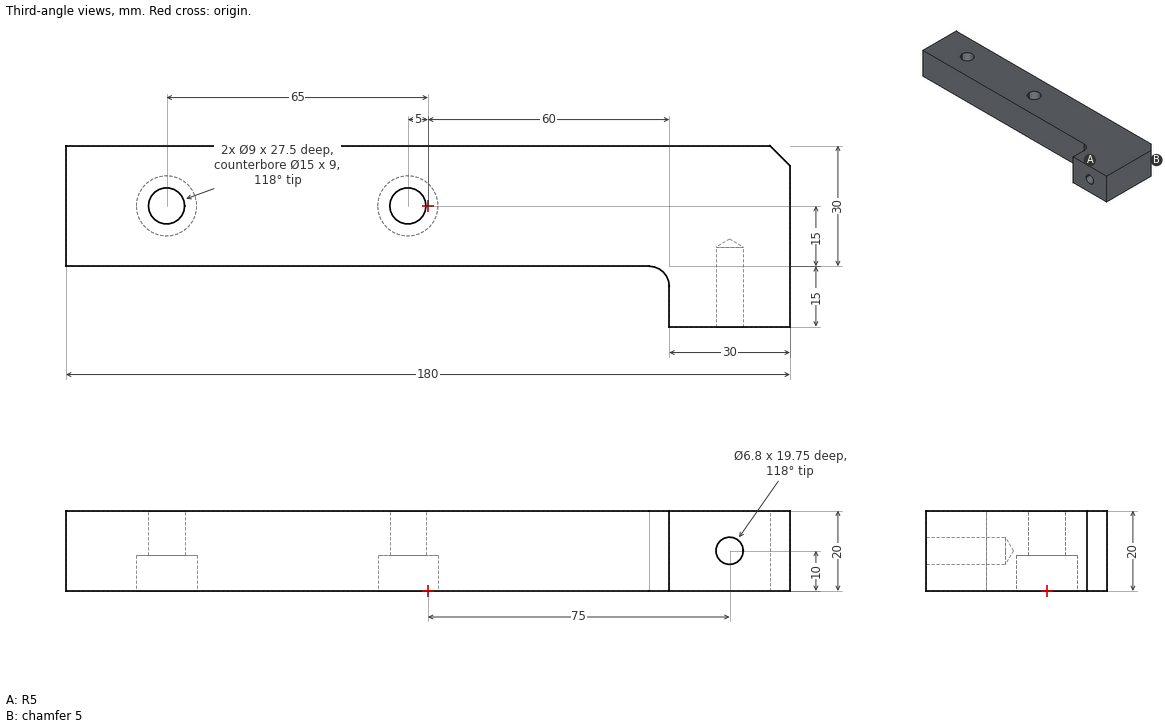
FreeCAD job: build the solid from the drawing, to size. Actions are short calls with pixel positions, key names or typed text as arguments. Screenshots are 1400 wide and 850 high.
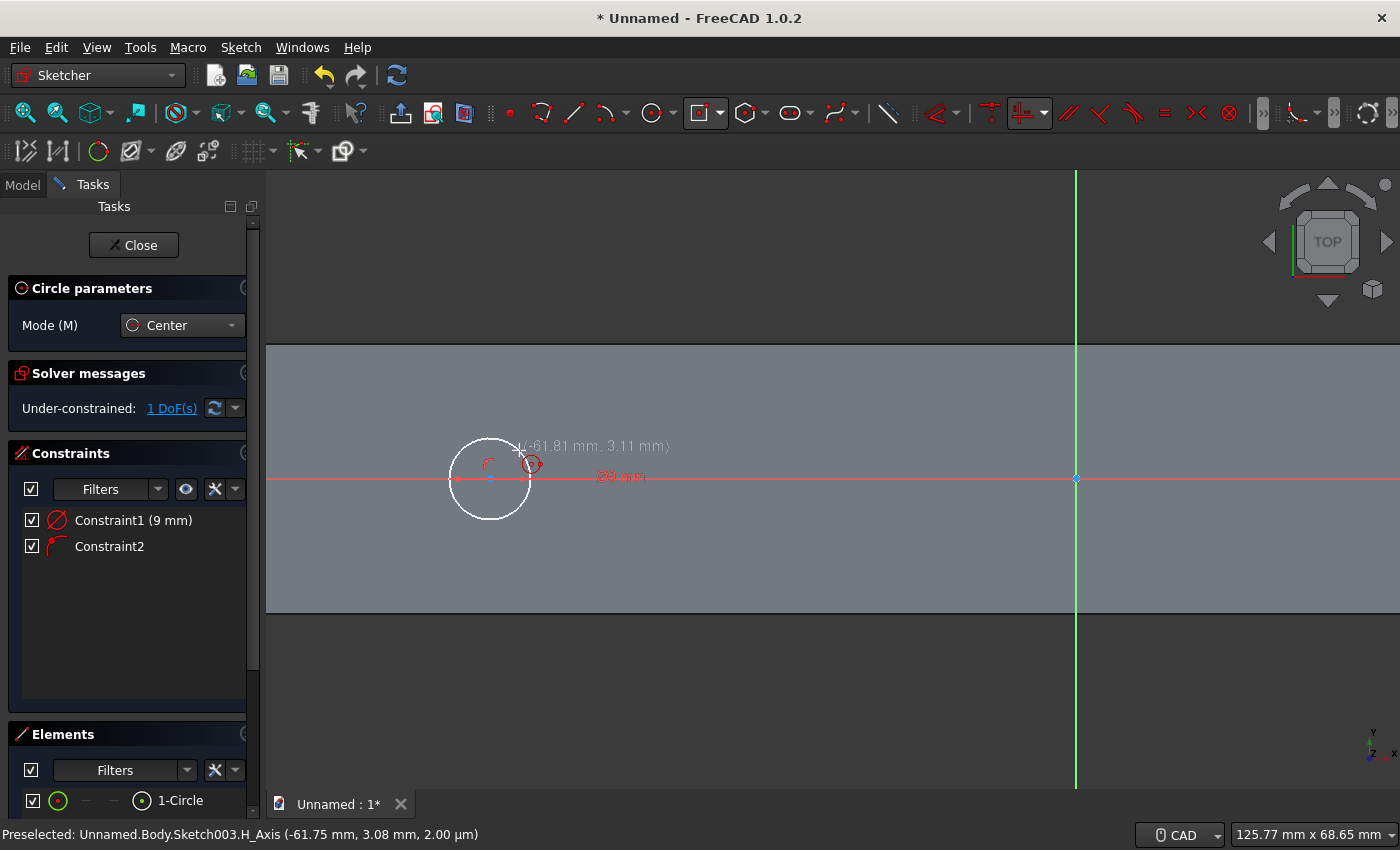
click(1031, 479)
move(1060, 450)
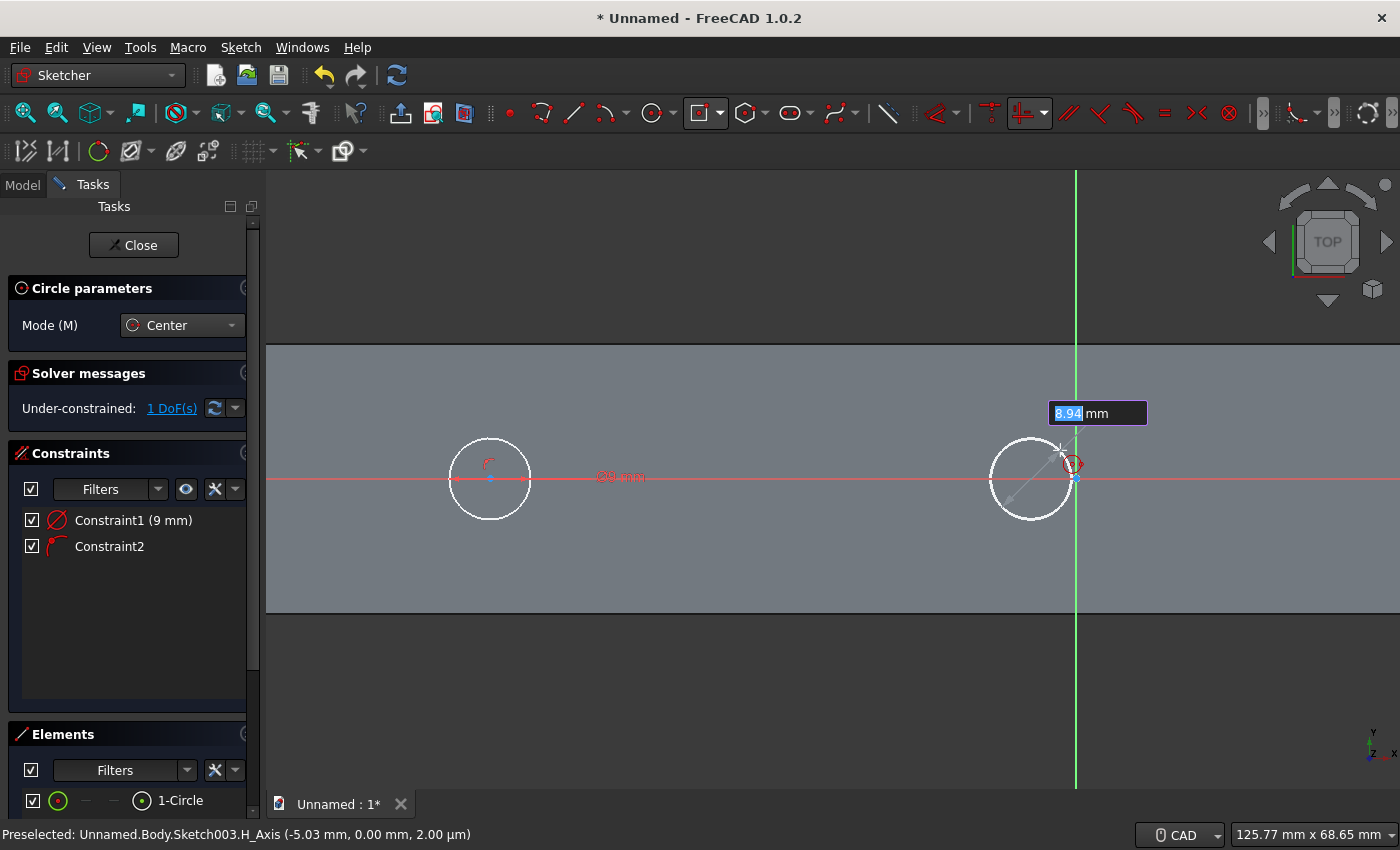
text(9)
key(Return)
key(Escape)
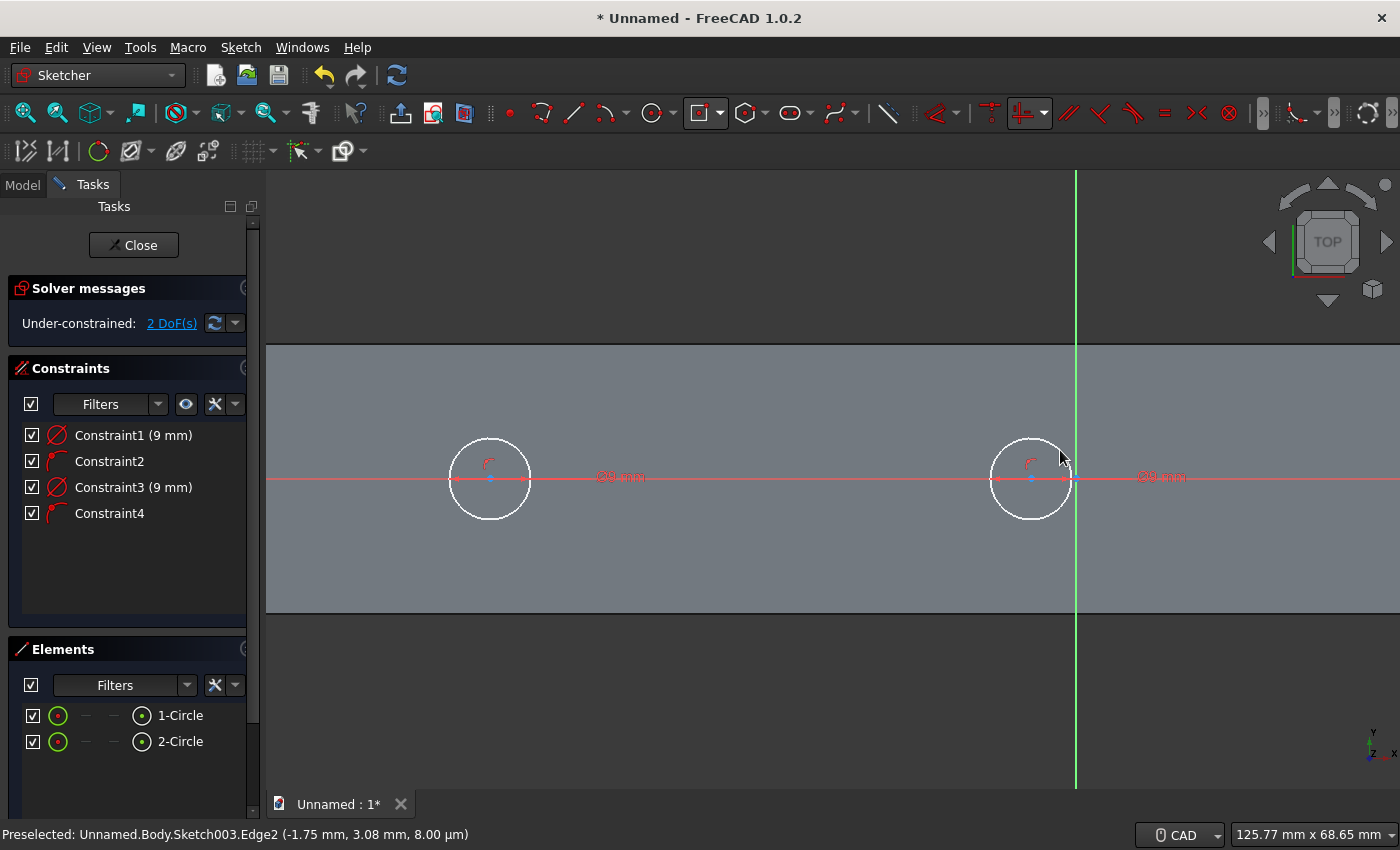
click(936, 114)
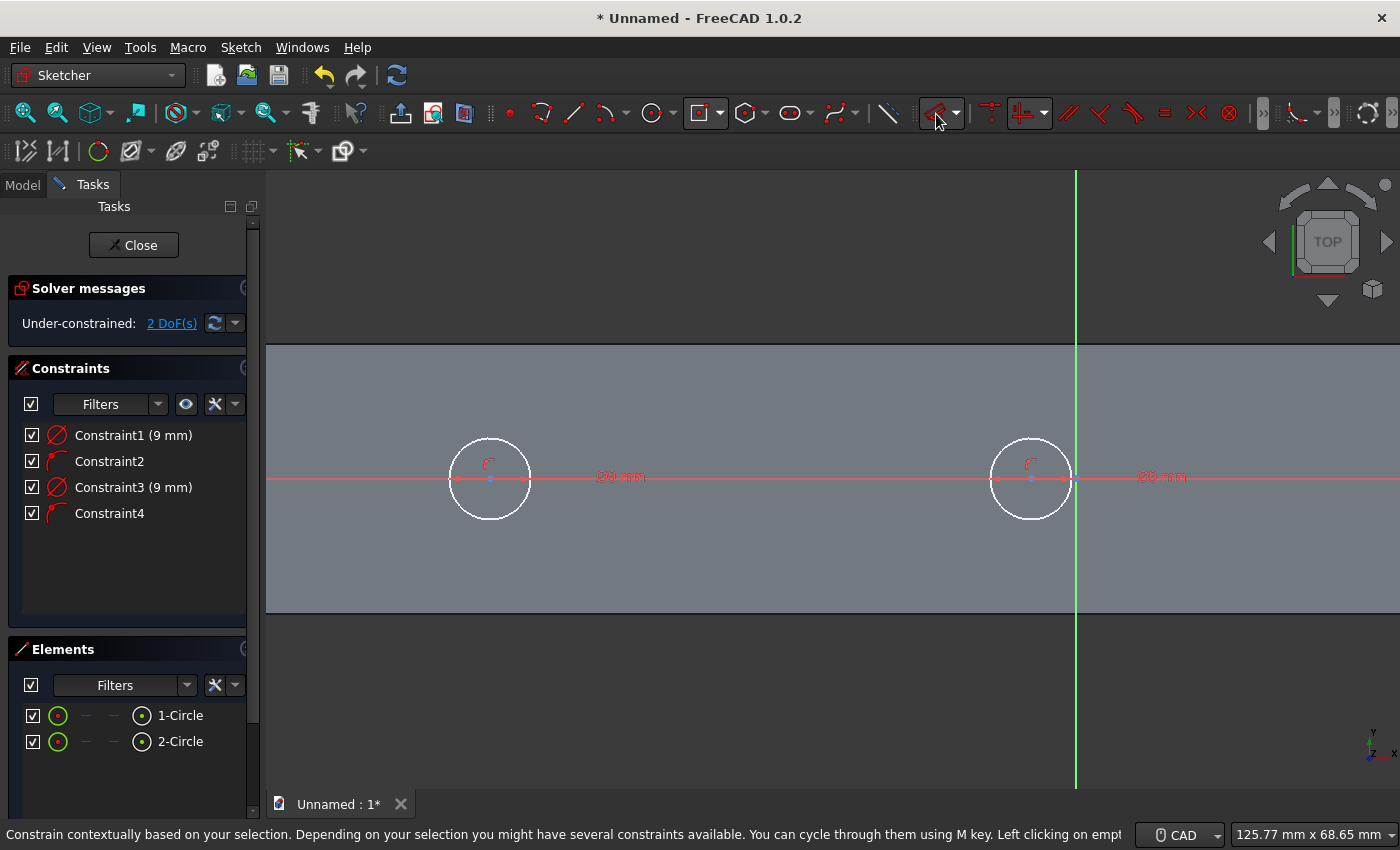
click(1031, 479)
click(1054, 537)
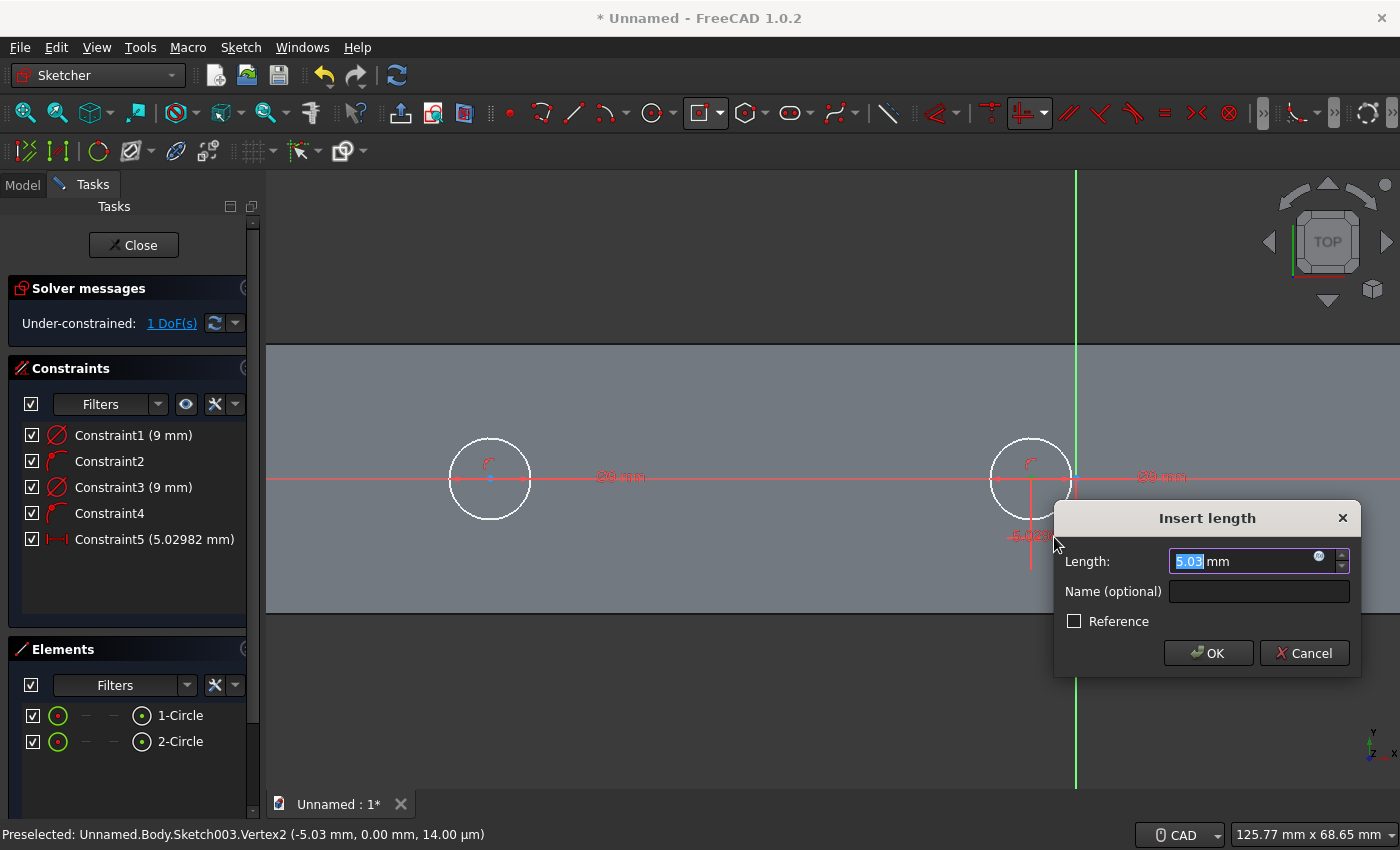
text(5)
key(Return)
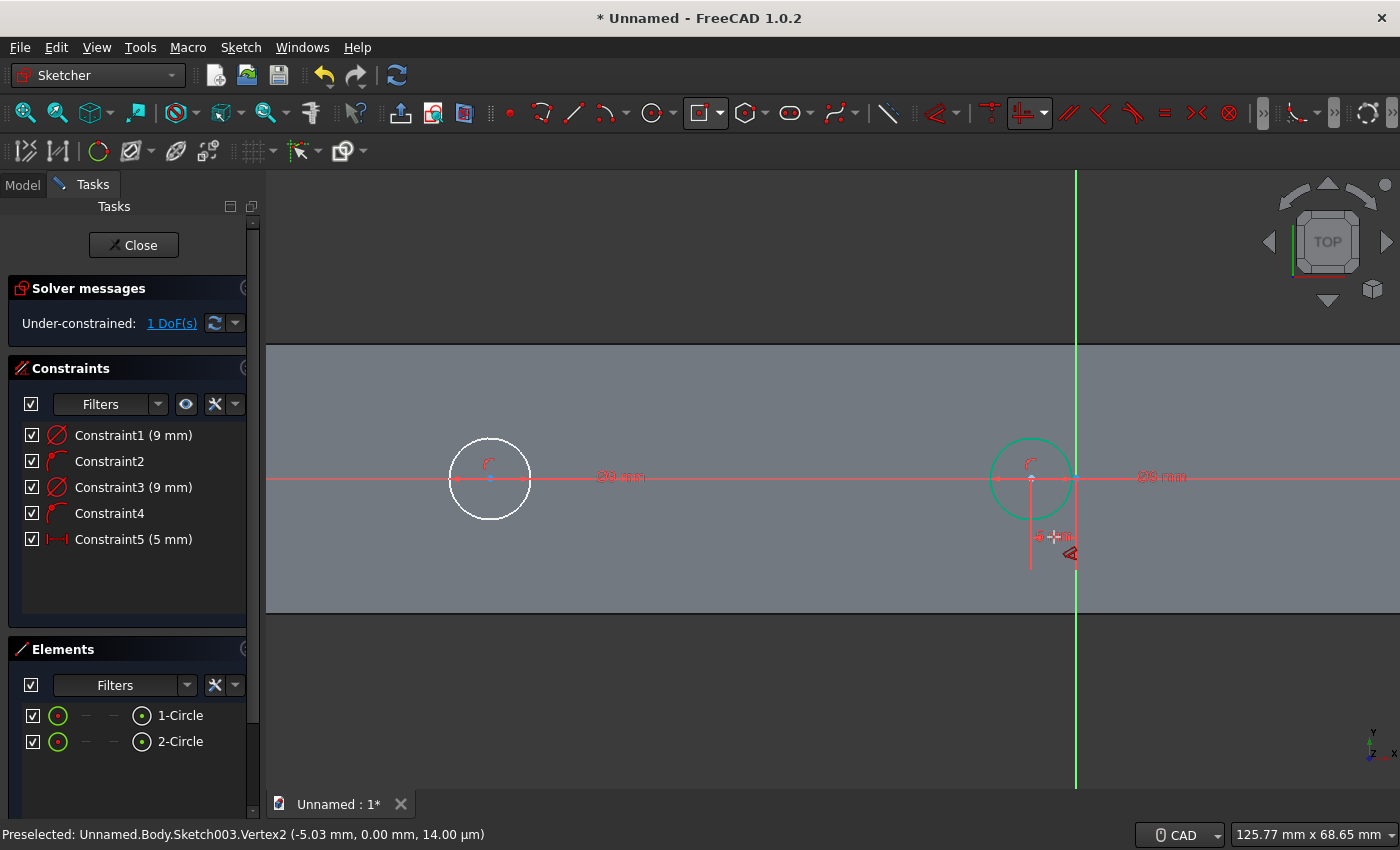
click(490, 479)
click(783, 513)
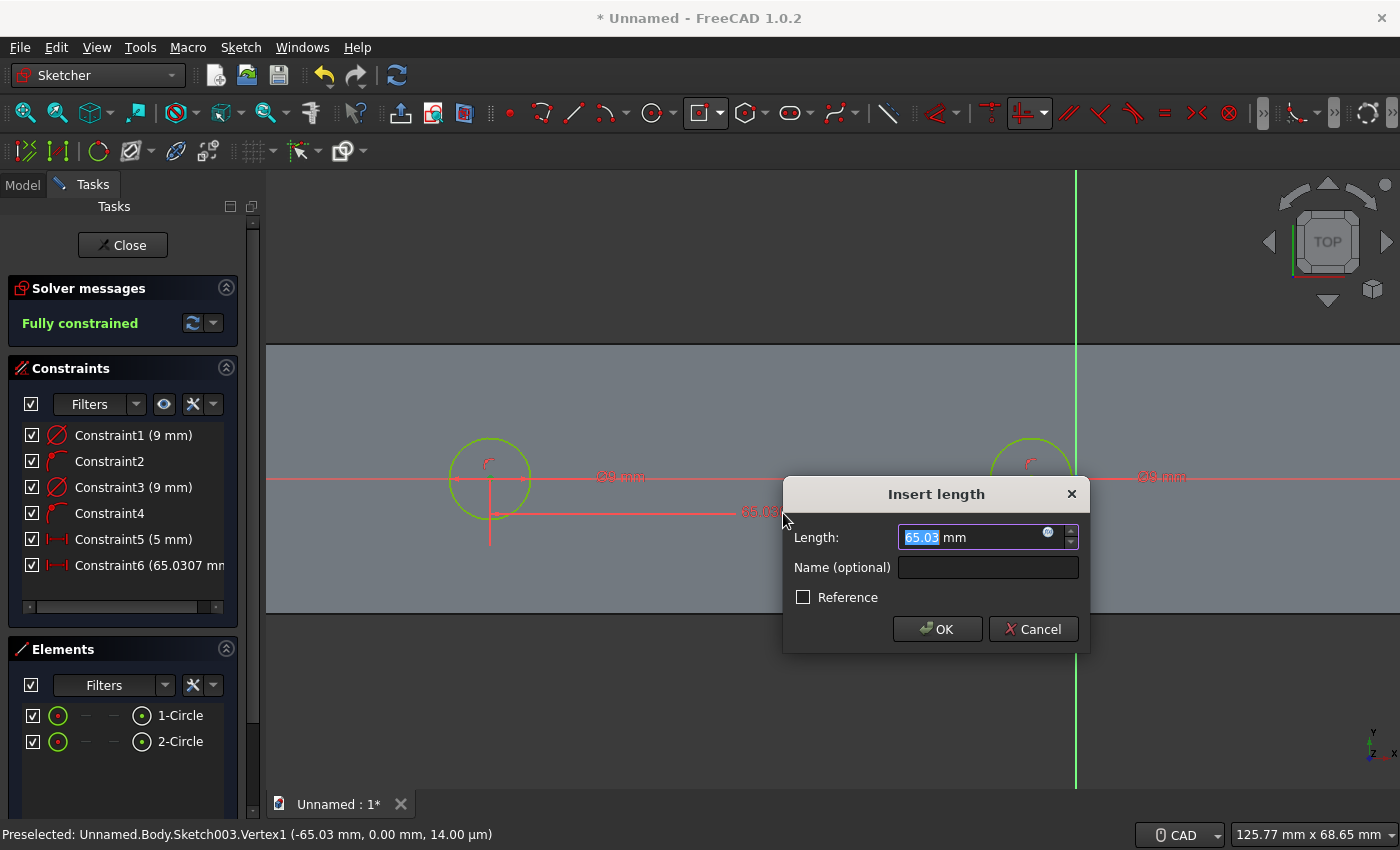
text(65)
key(Return)
key(Escape)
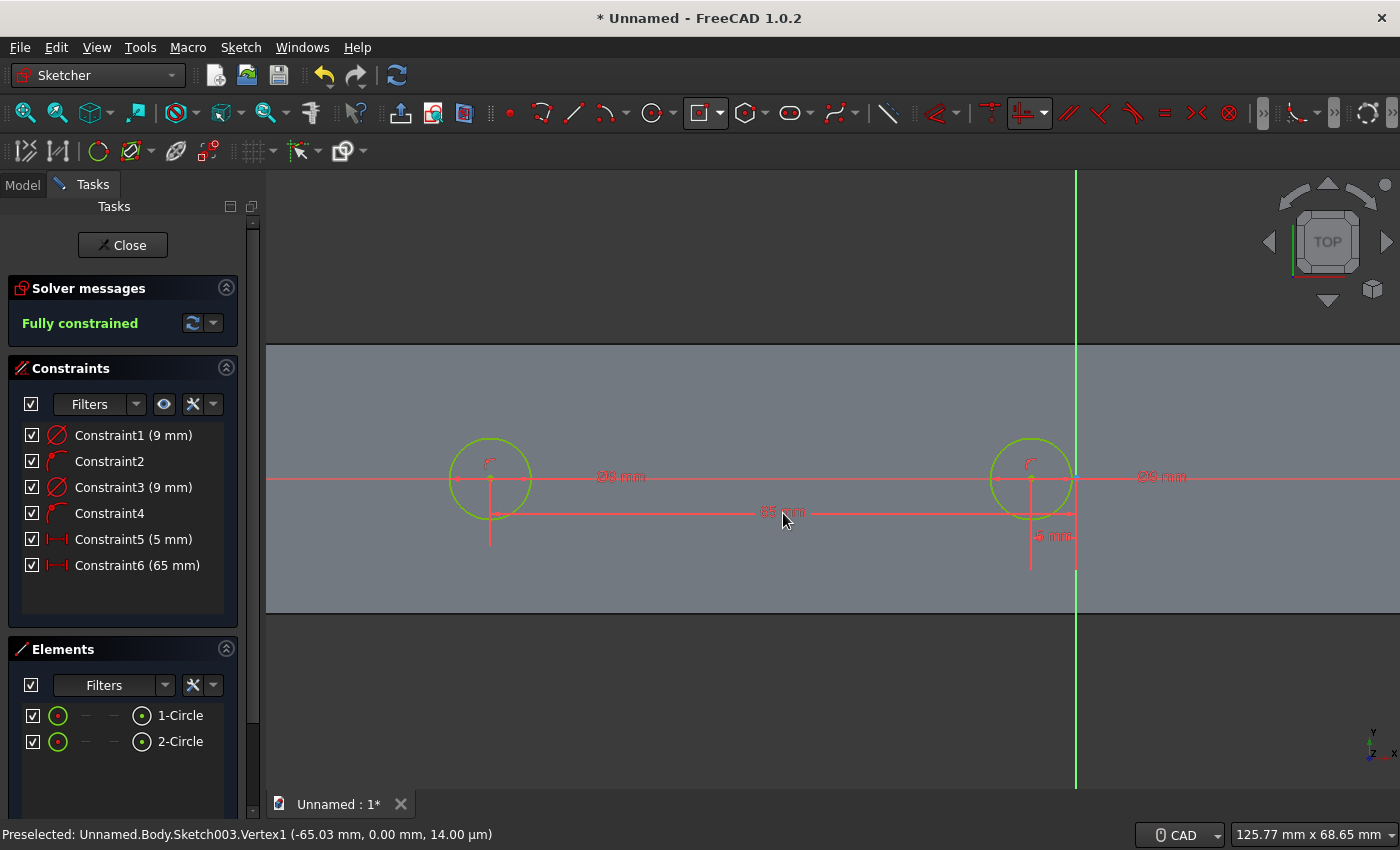
click(123, 245)